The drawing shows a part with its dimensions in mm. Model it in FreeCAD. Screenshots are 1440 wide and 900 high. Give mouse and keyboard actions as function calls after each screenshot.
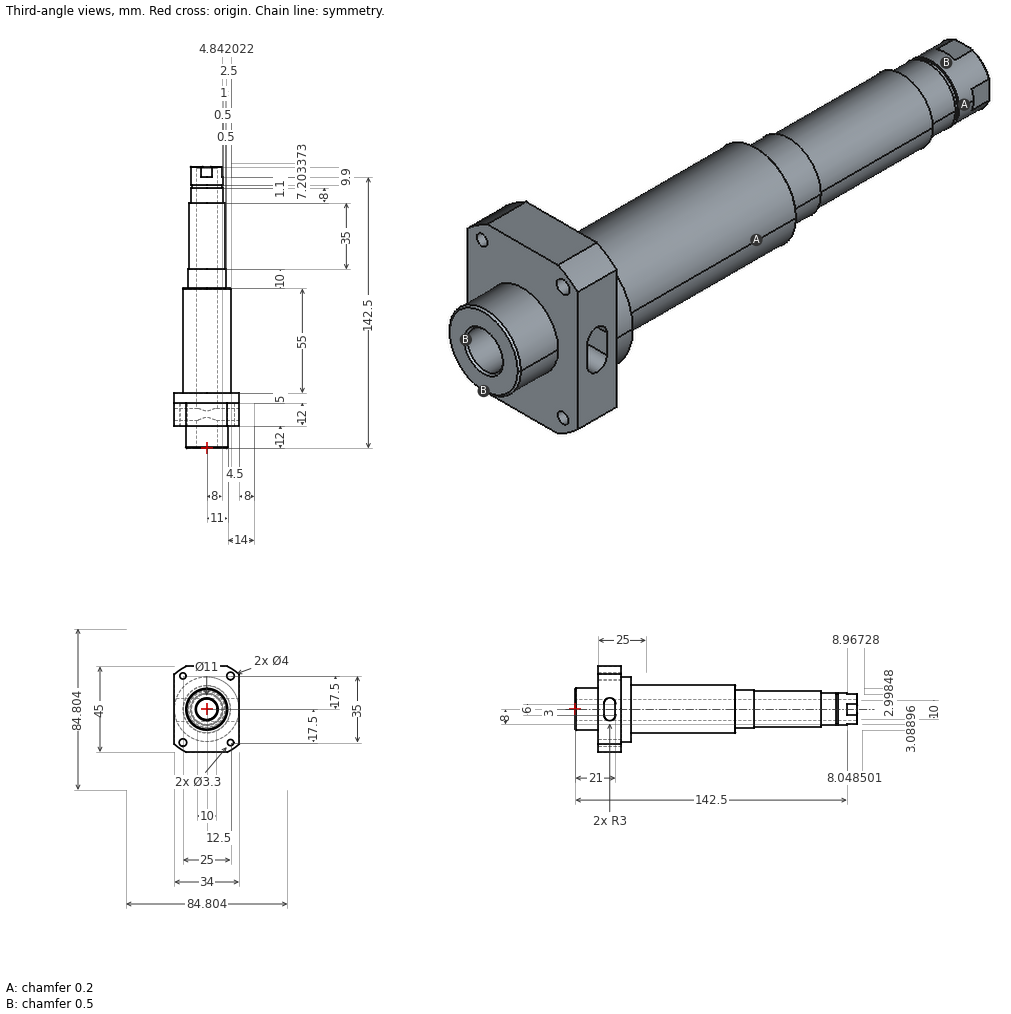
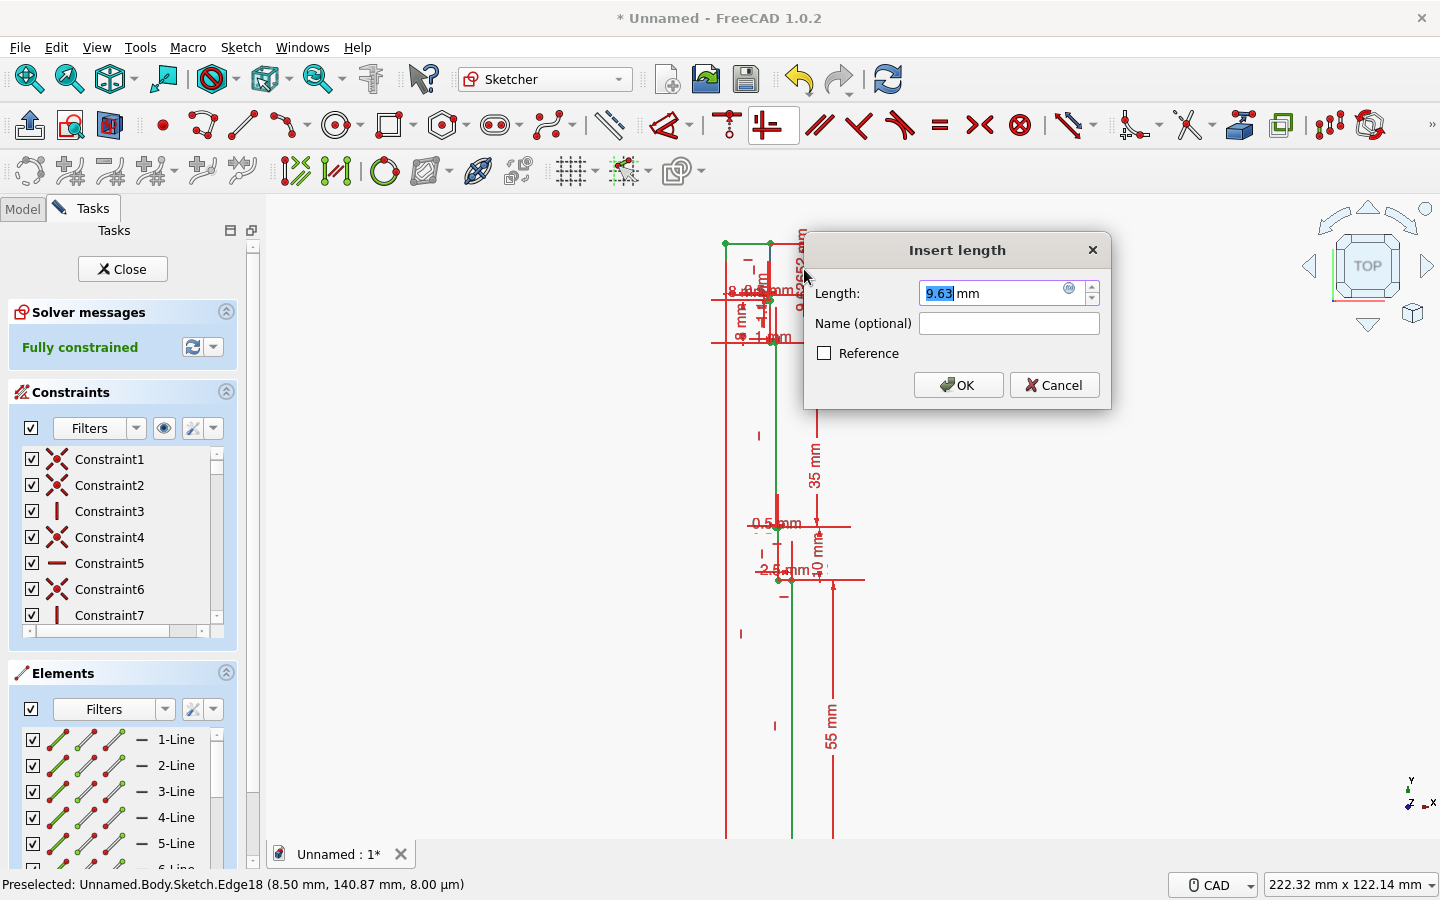
text(9.9)
key(Return)
key(Escape)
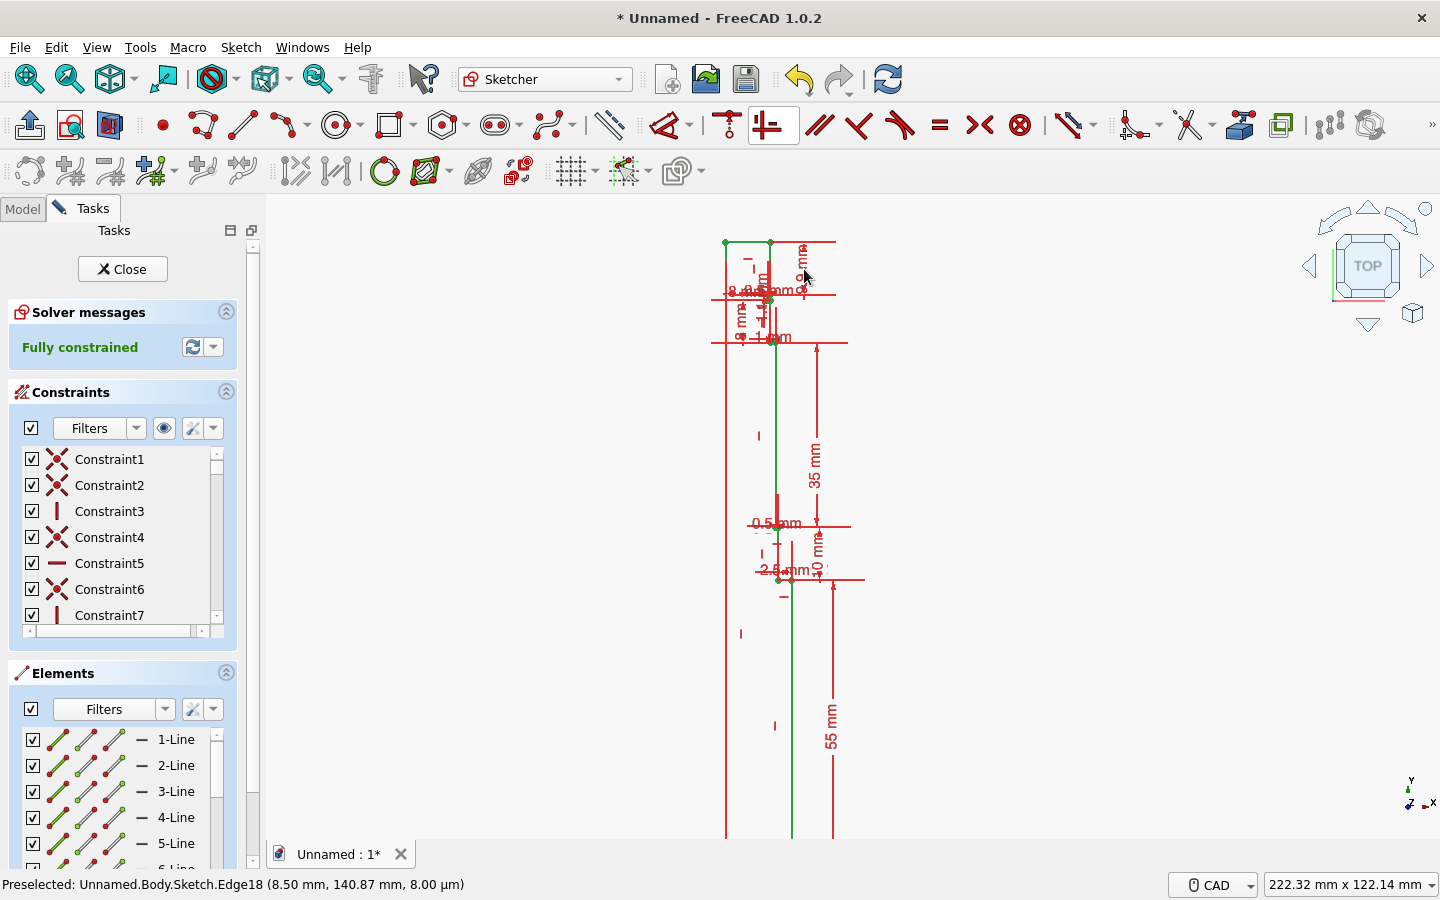
click(123, 269)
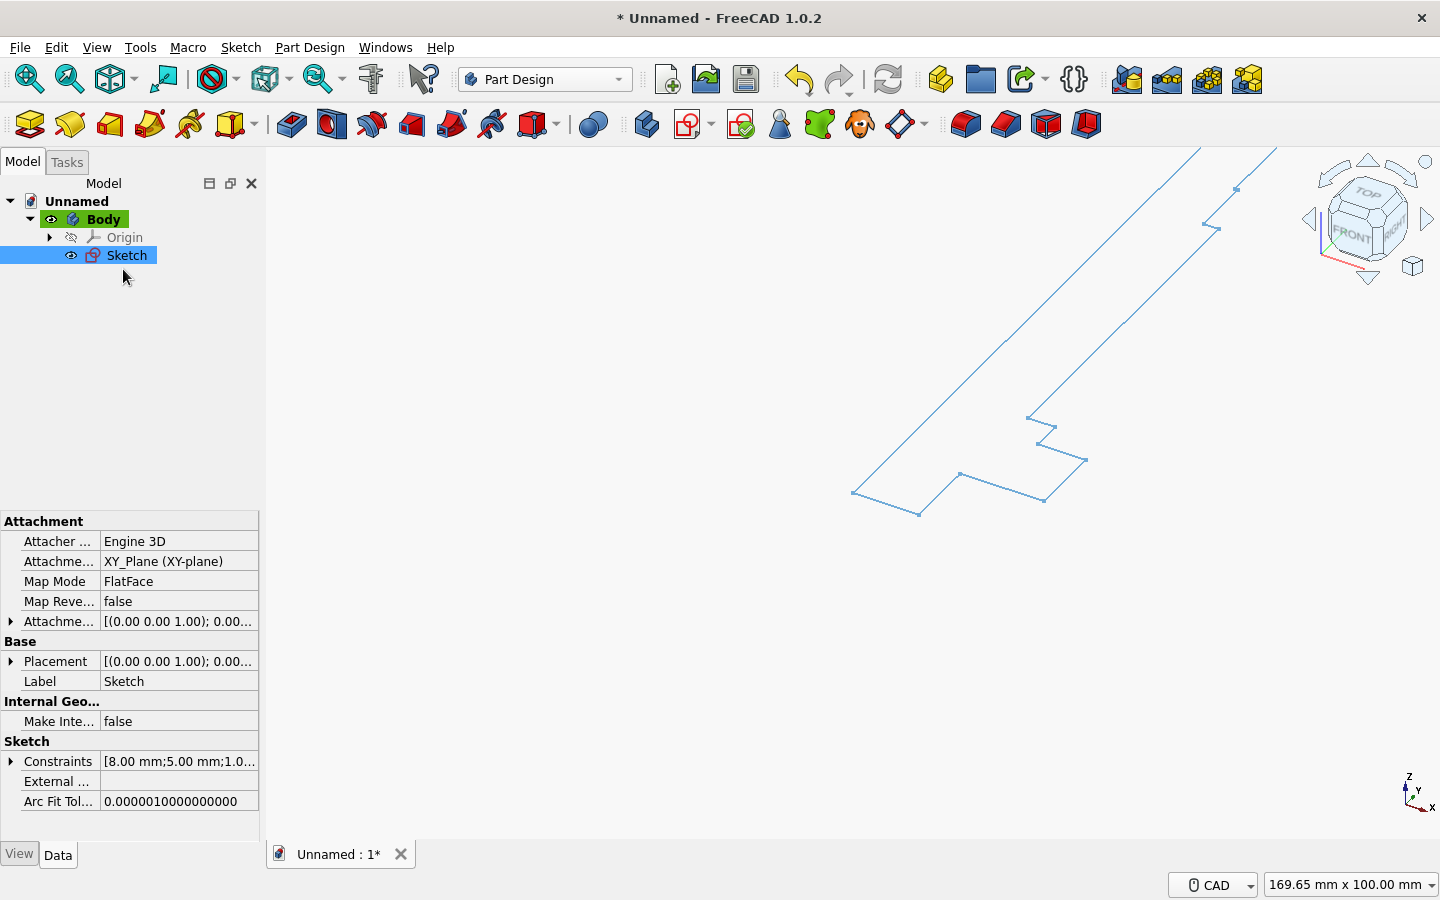
click(70, 124)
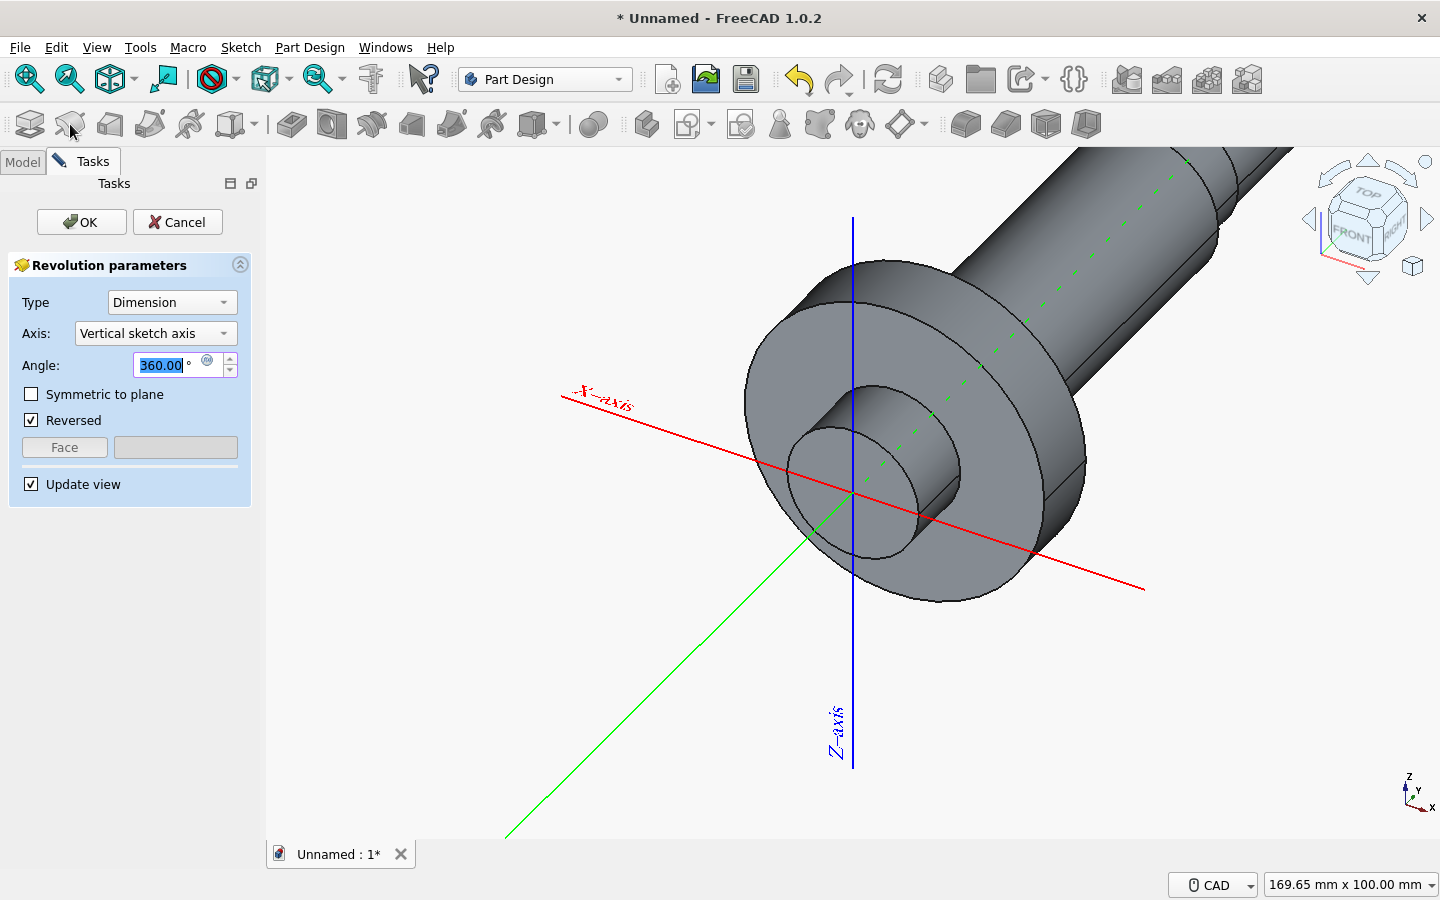
click(82, 222)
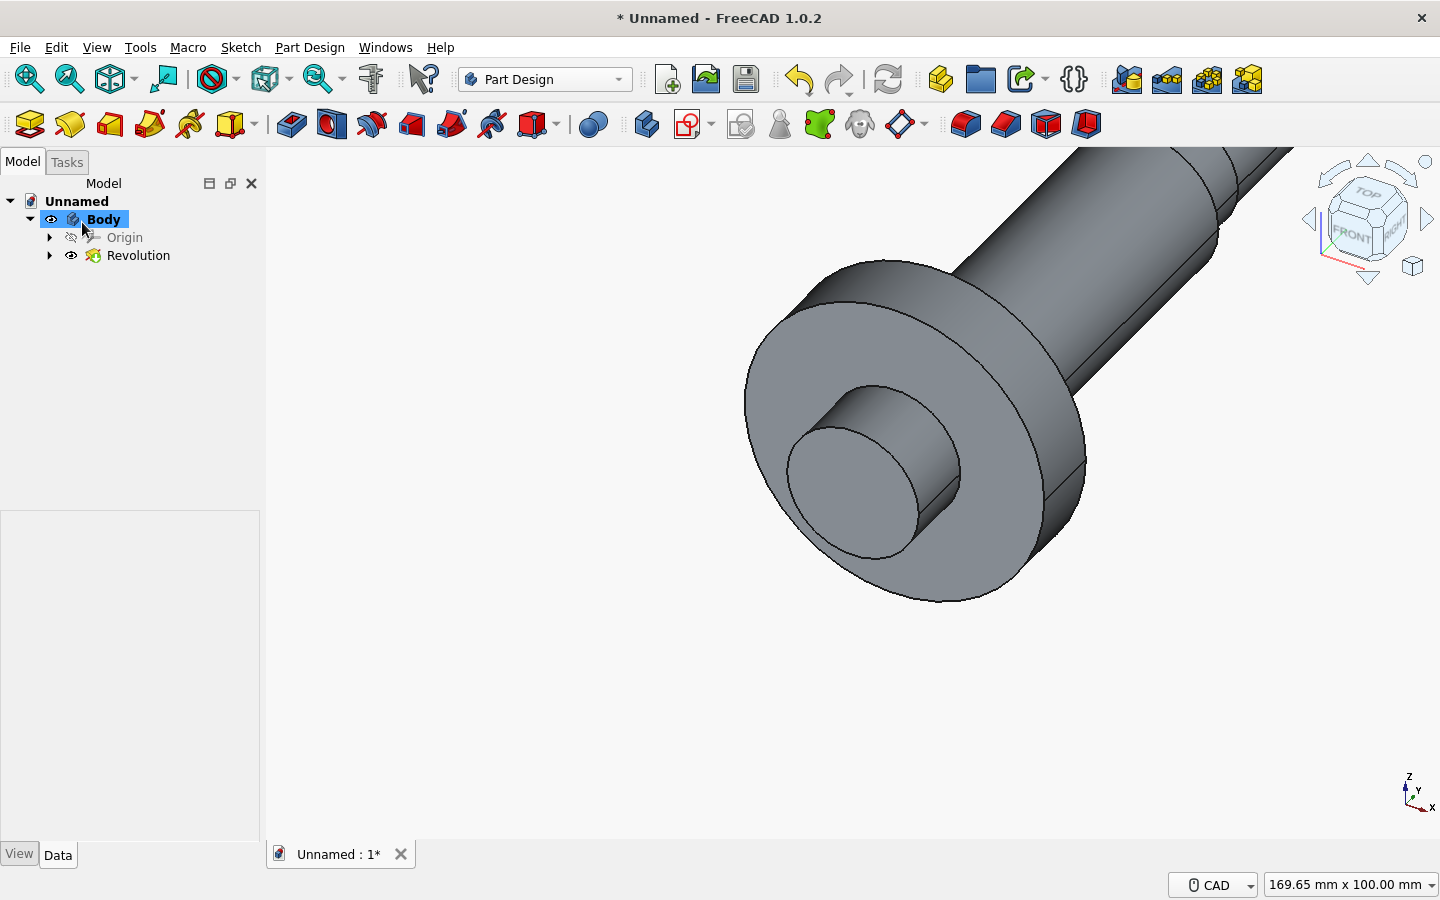
click(30, 80)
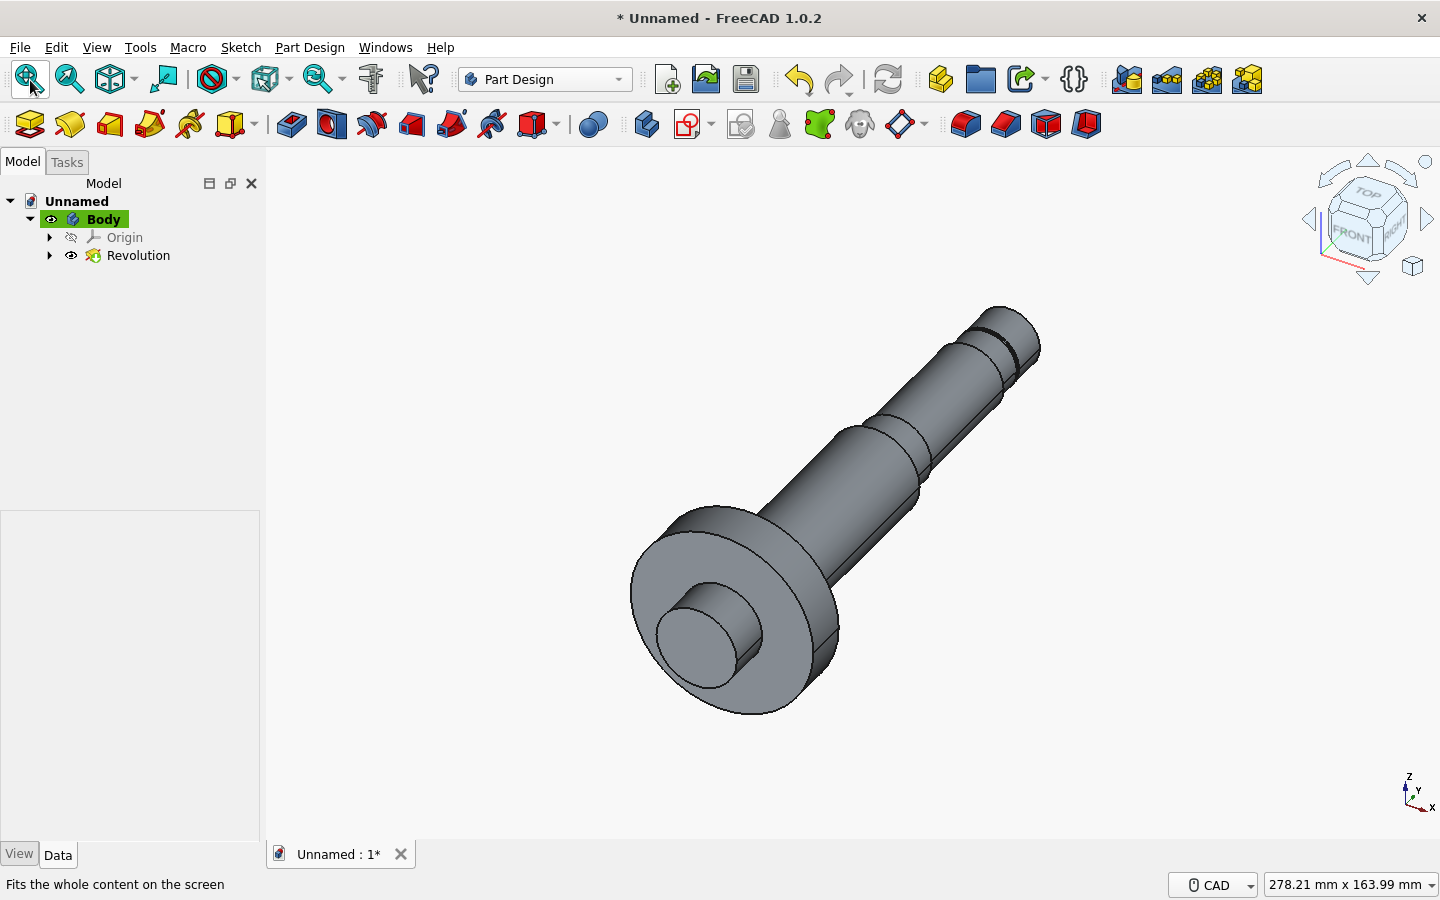
key(4)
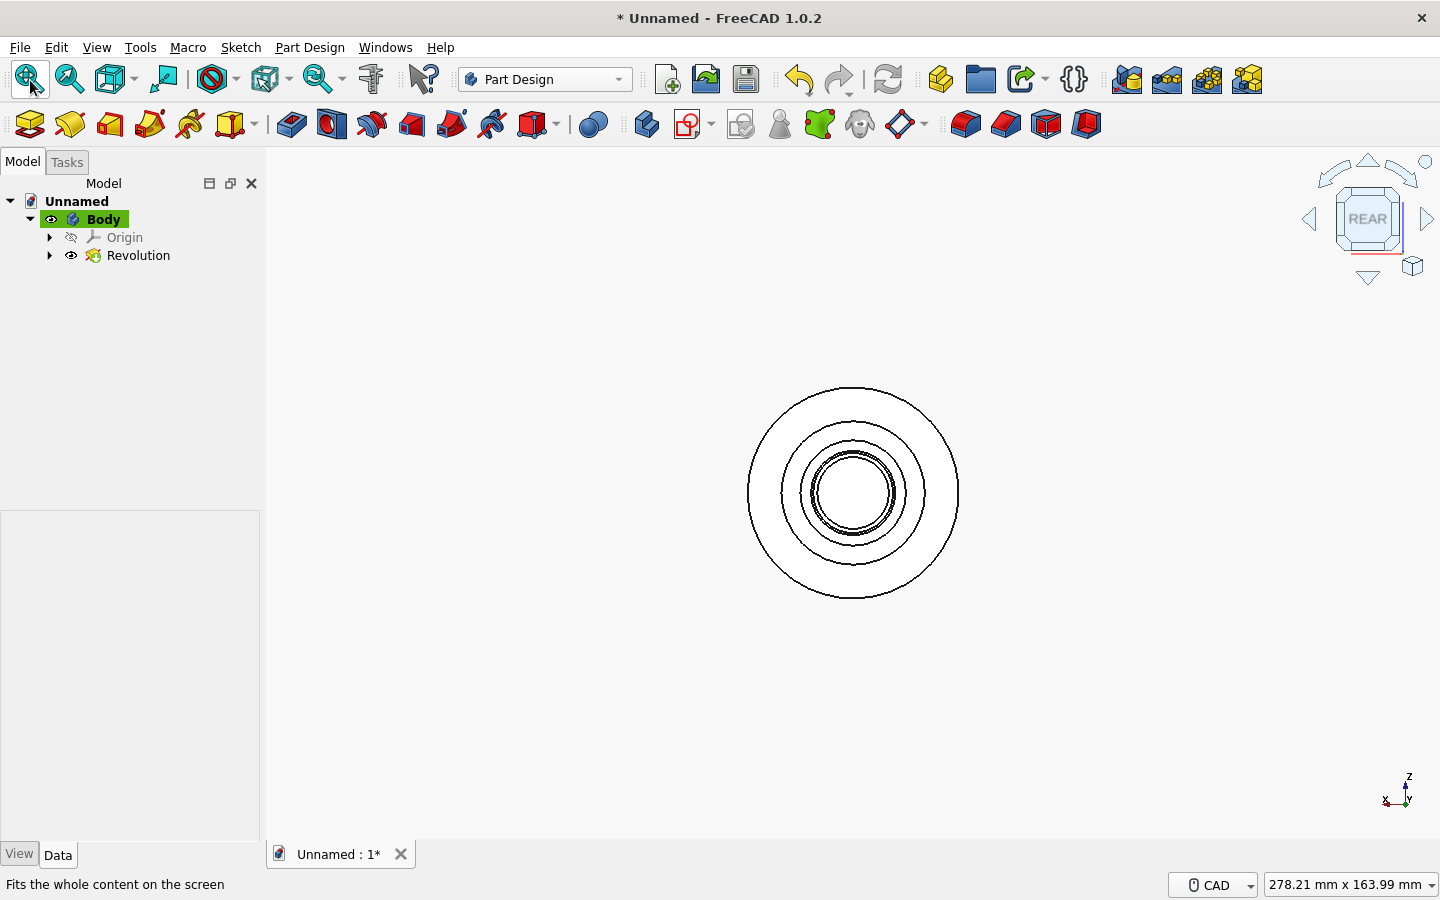
click(30, 80)